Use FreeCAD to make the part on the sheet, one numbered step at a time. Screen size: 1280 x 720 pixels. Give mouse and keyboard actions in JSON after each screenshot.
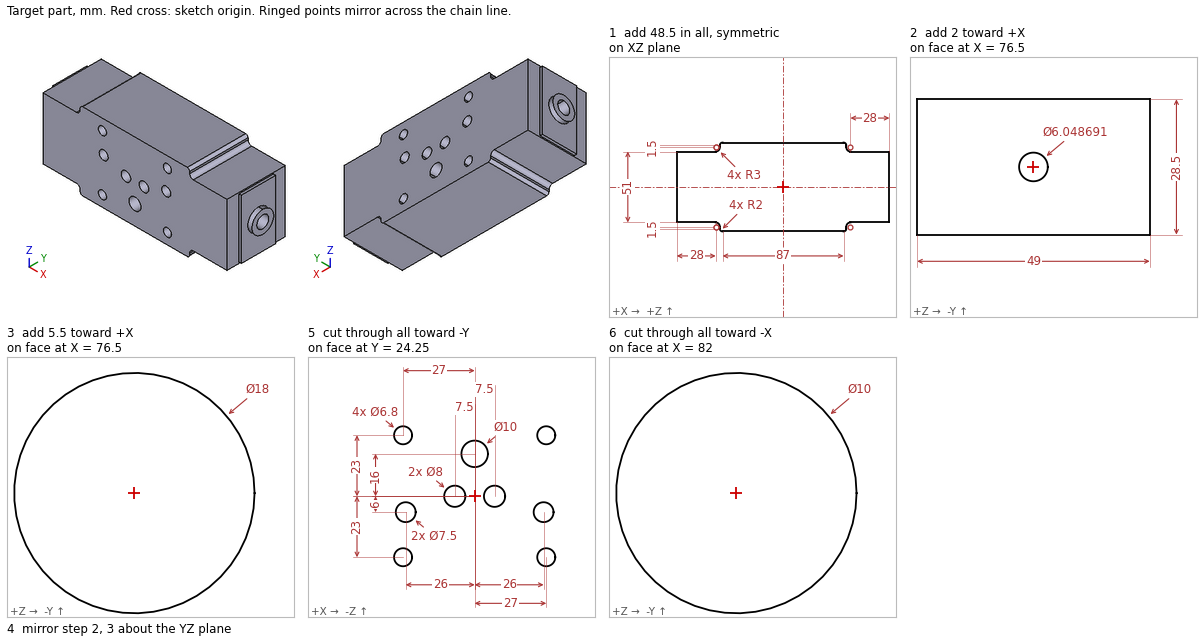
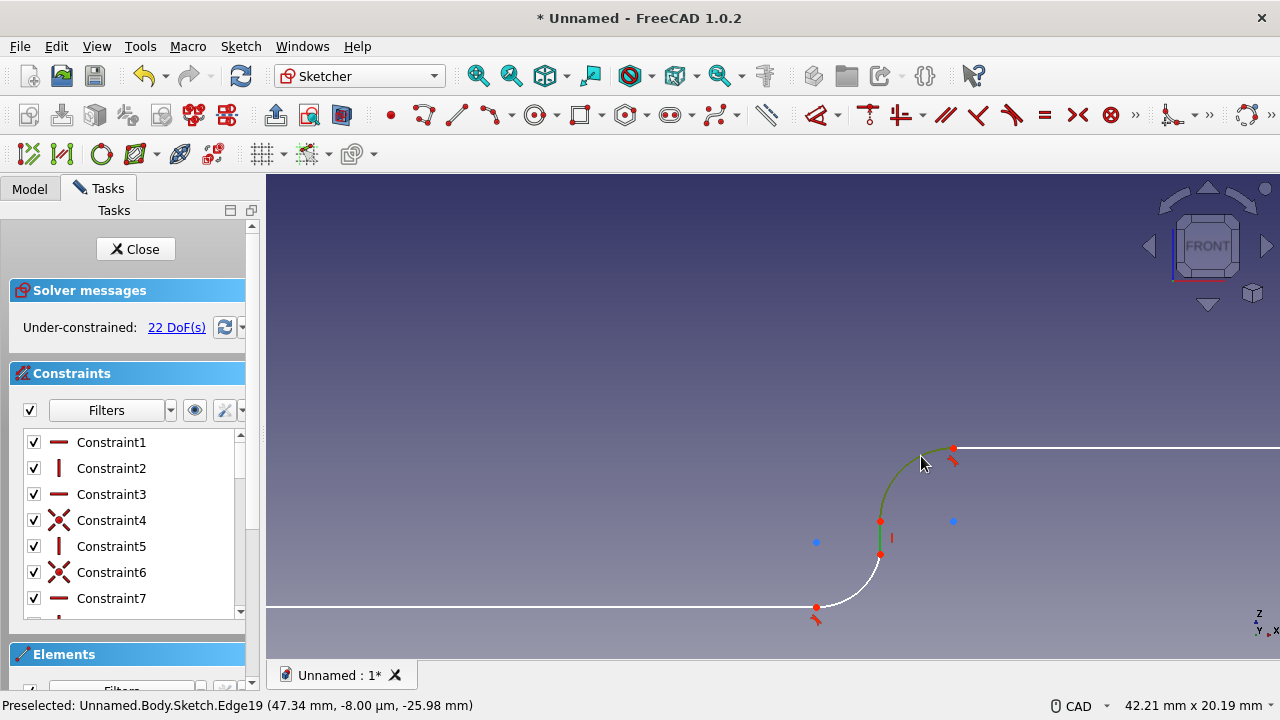
{"action": "key", "text": "t"}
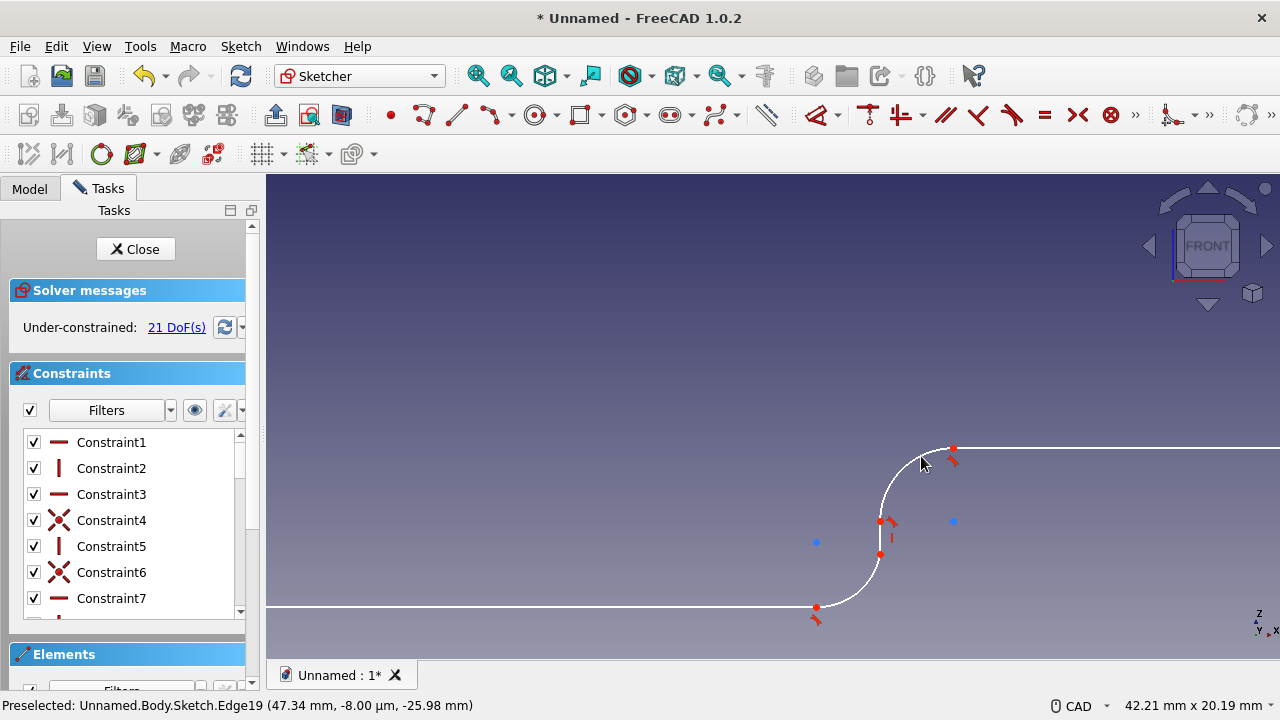
{"action": "scroll", "coordinate": [880, 531], "scroll_direction": "up", "scroll_amount": 2}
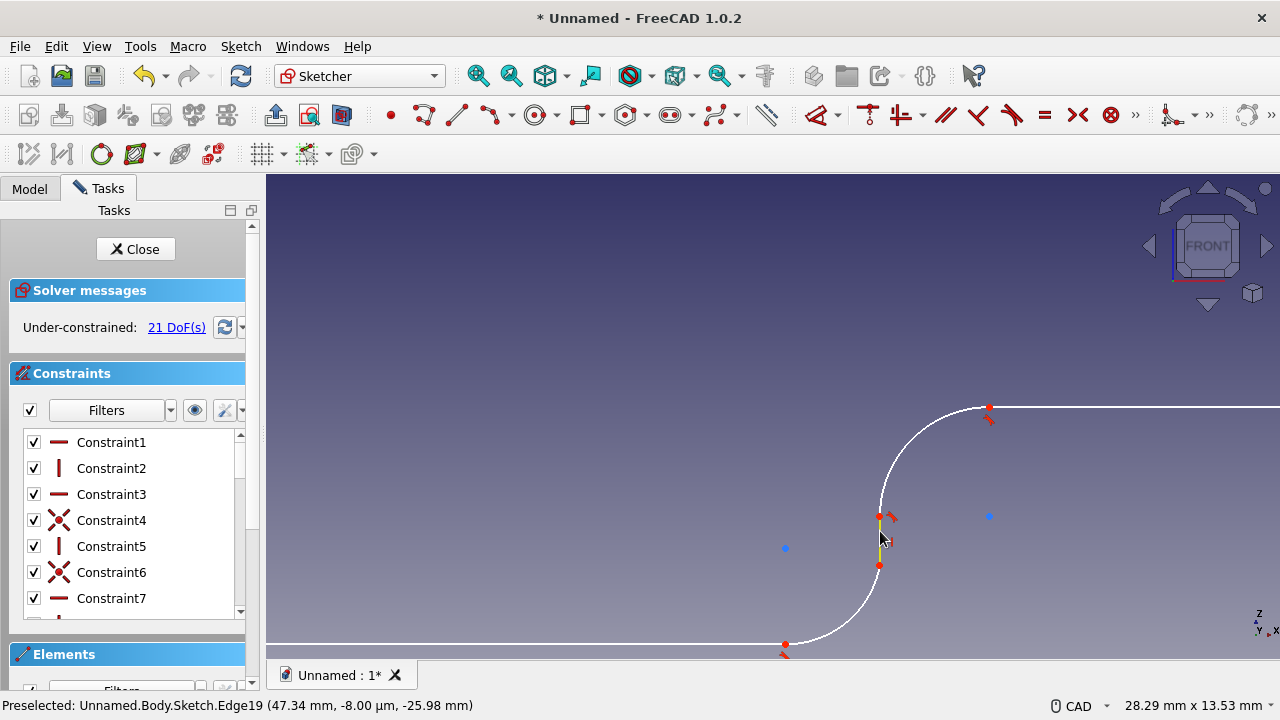
{"action": "left_click", "coordinate": [880, 531]}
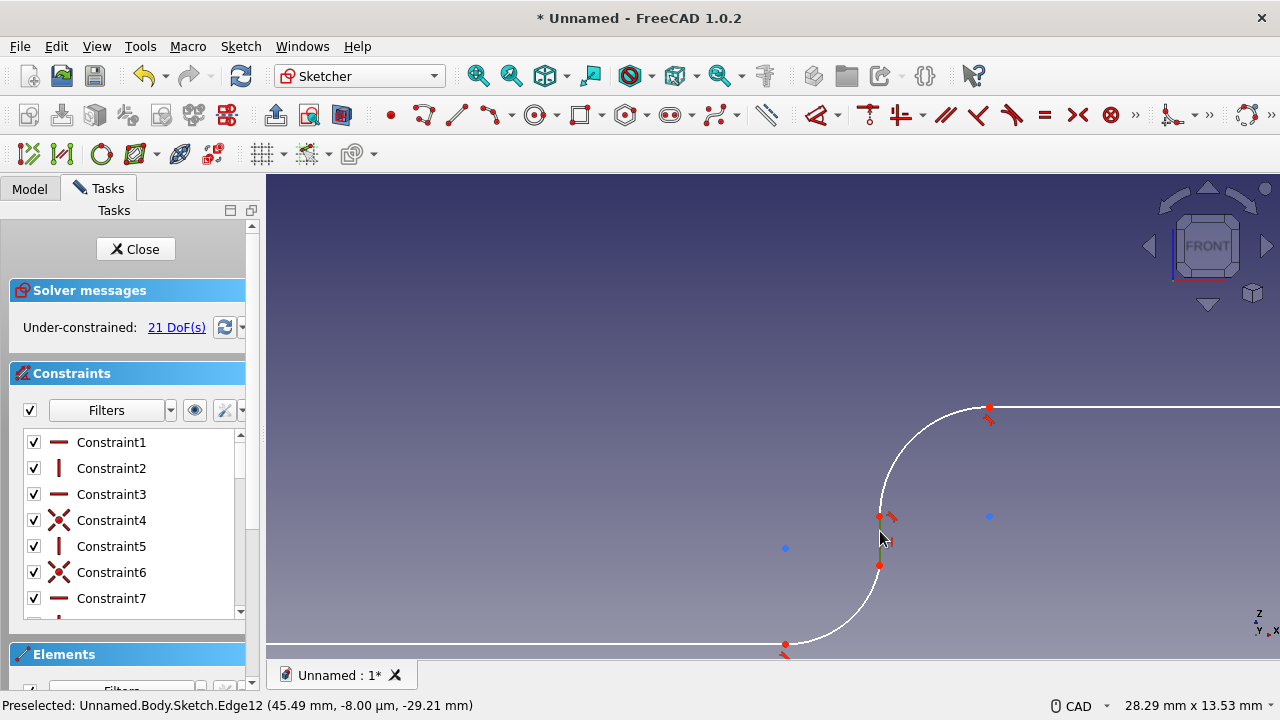
{"action": "scroll", "coordinate": [886, 533], "scroll_direction": "down", "scroll_amount": 11}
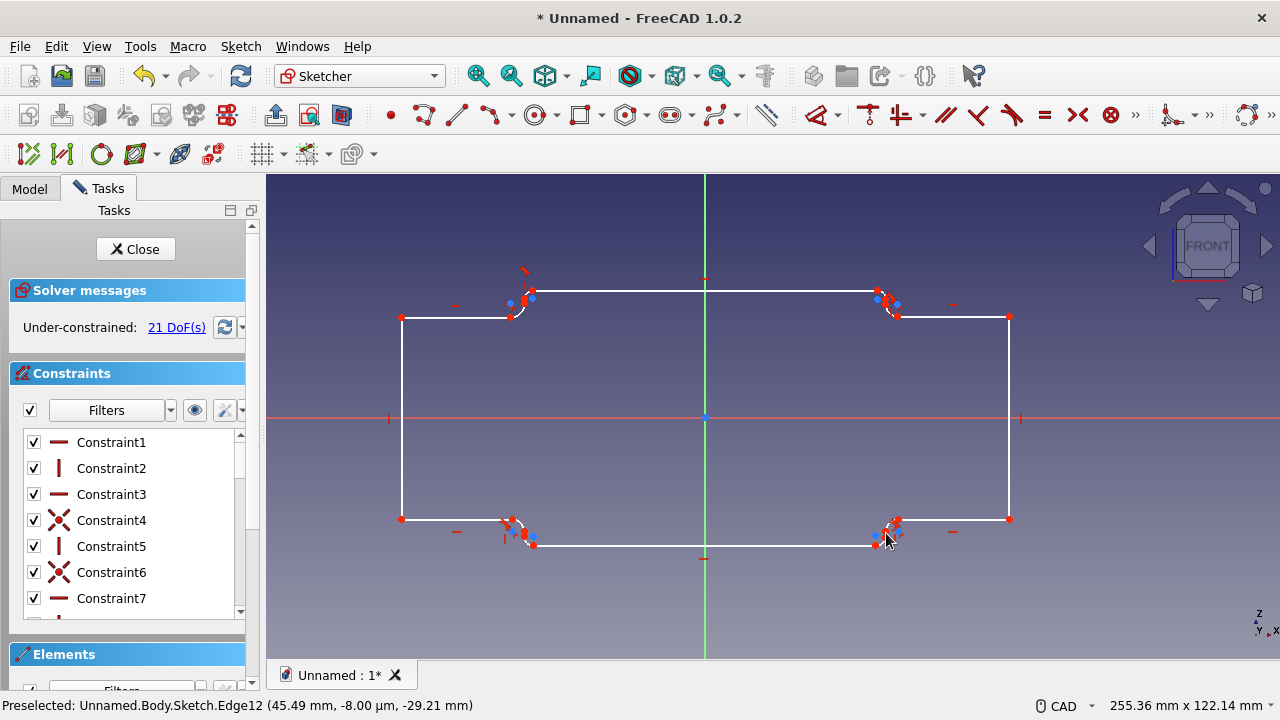
{"action": "scroll", "coordinate": [884, 541], "scroll_direction": "up", "scroll_amount": 6}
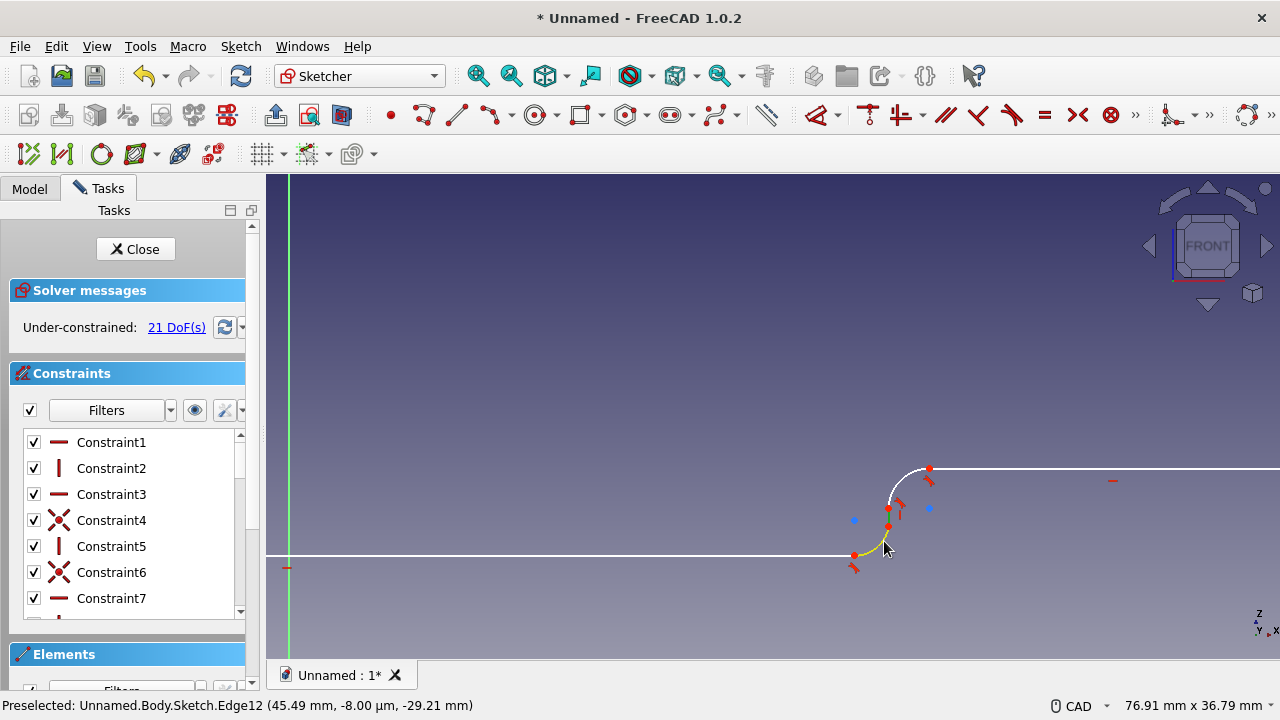
{"action": "left_click", "coordinate": [883, 540]}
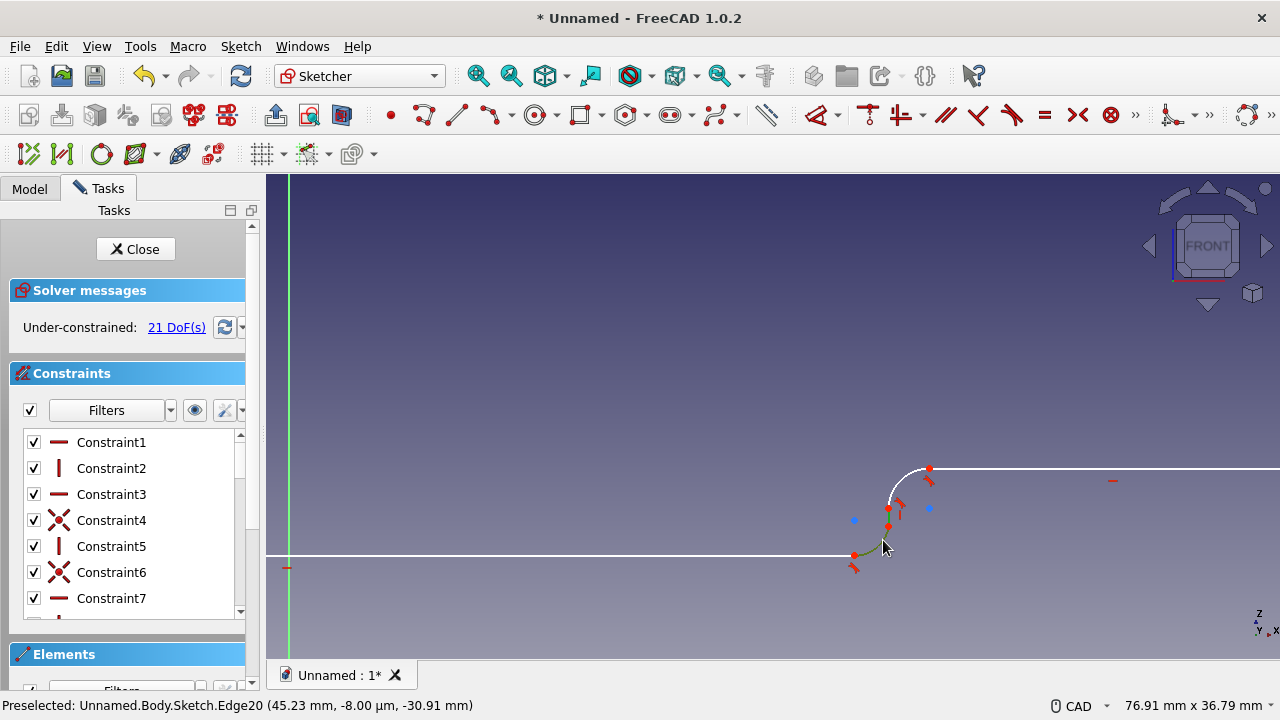
{"action": "left_click", "coordinate": [1012, 116]}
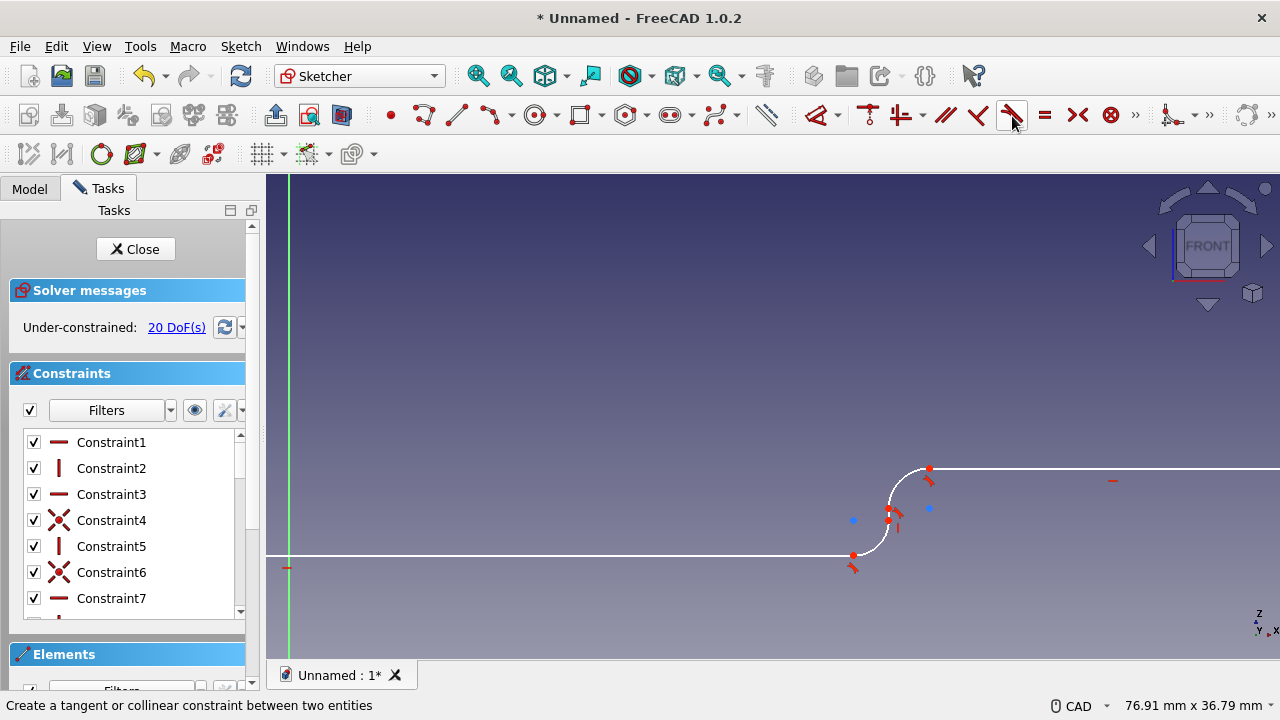
{"action": "scroll", "coordinate": [884, 540], "scroll_direction": "down", "scroll_amount": 6}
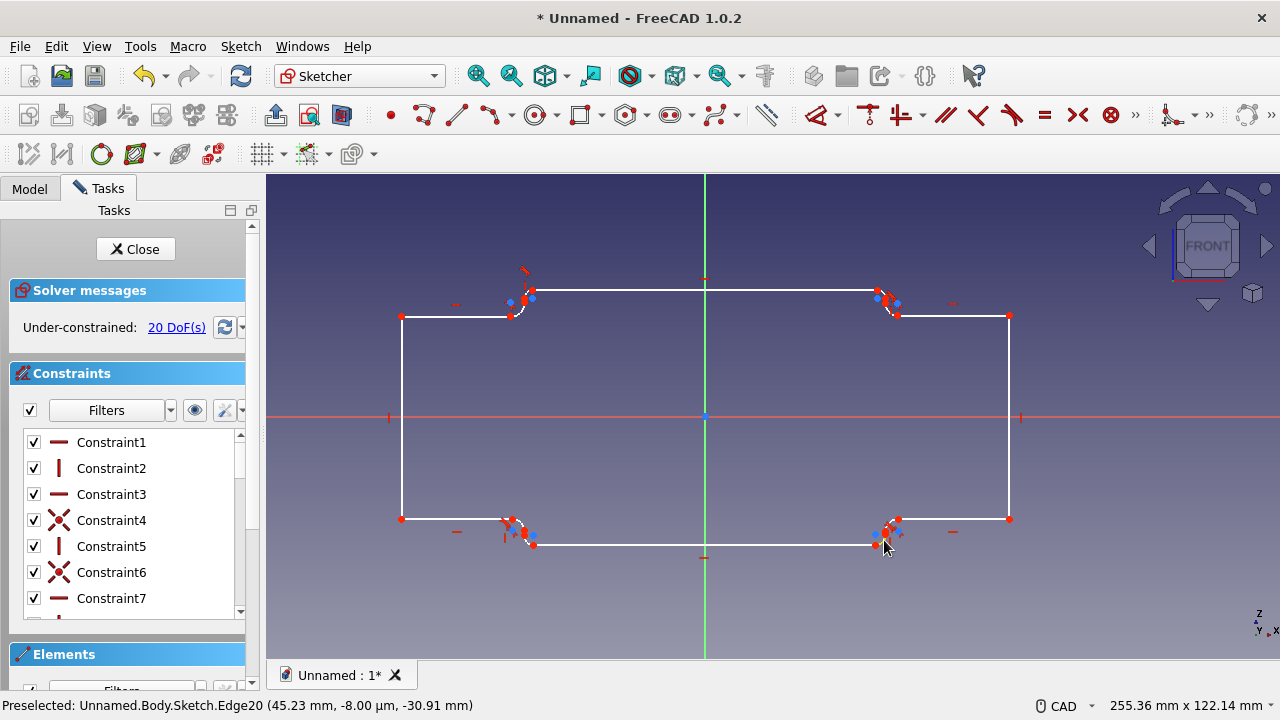
{"action": "scroll", "coordinate": [523, 525], "scroll_direction": "up", "scroll_amount": 5}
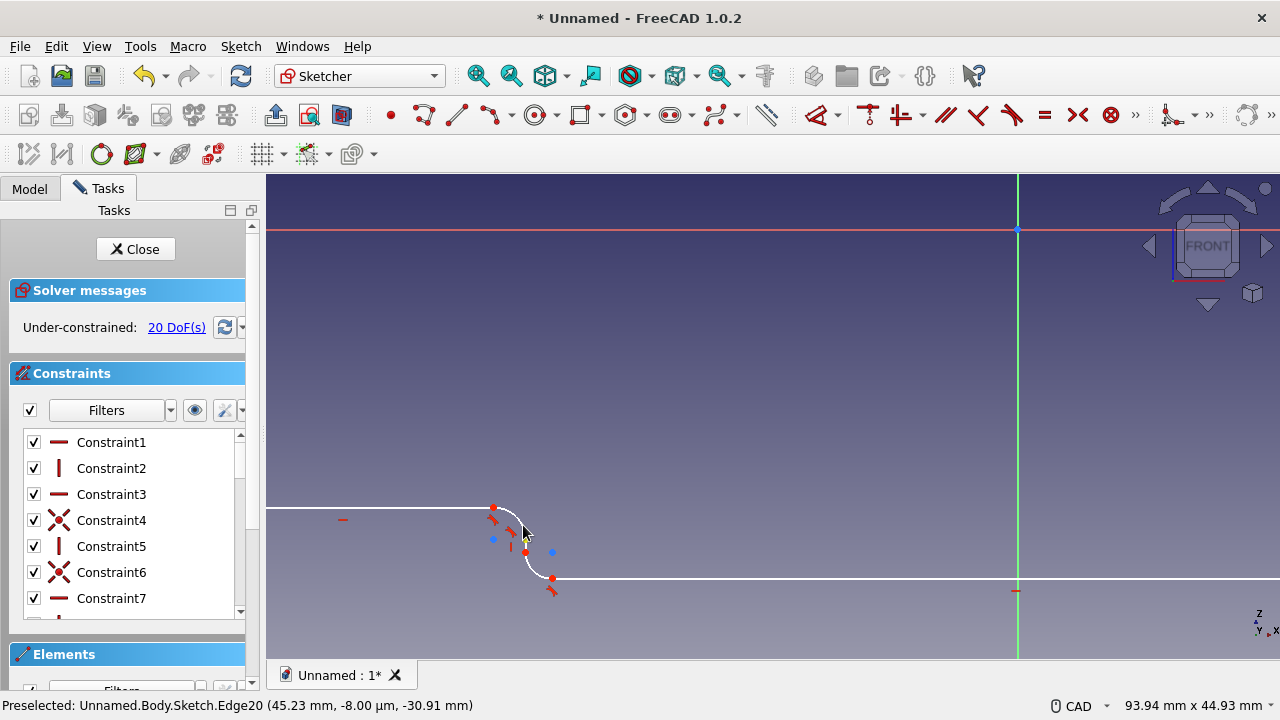
{"action": "left_click", "coordinate": [522, 525]}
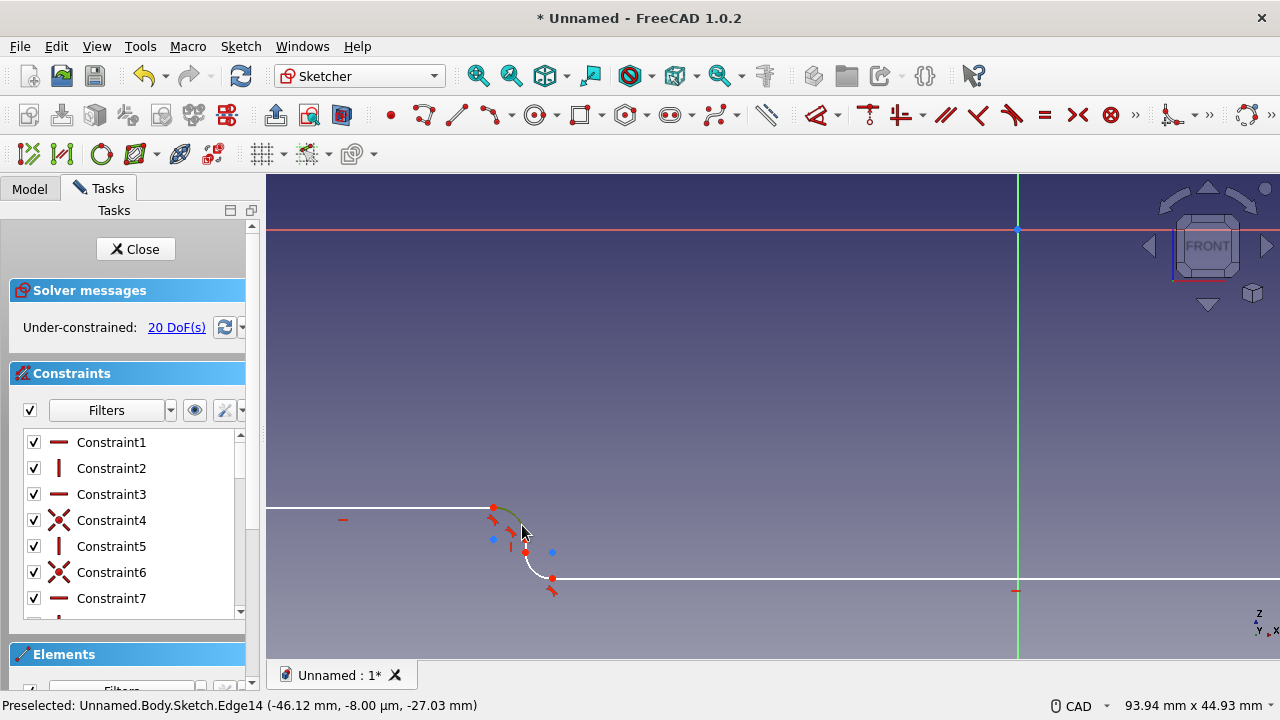
{"action": "scroll", "coordinate": [522, 525], "scroll_direction": "down", "scroll_amount": 5}